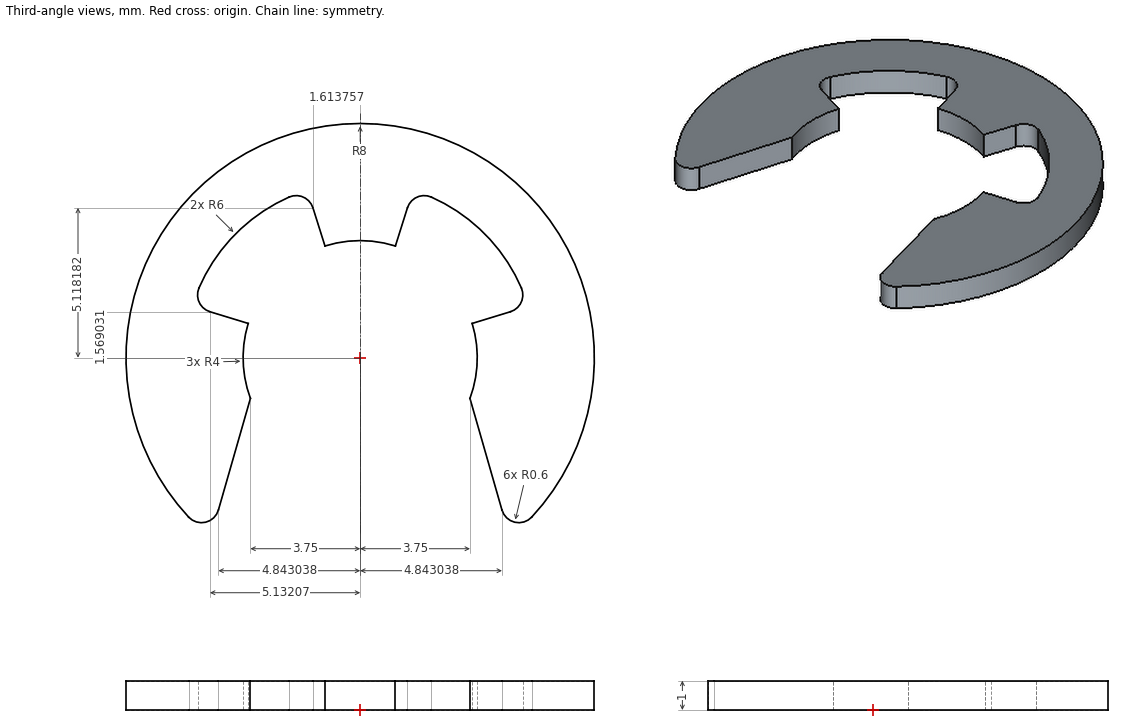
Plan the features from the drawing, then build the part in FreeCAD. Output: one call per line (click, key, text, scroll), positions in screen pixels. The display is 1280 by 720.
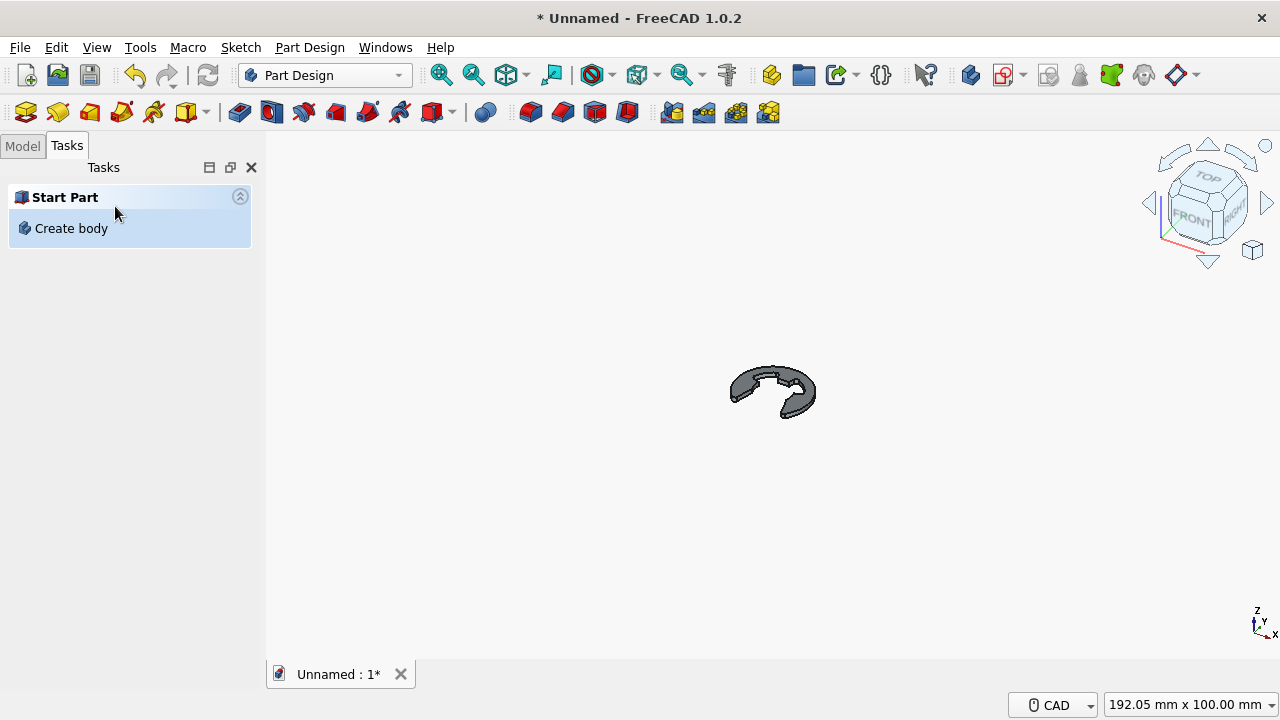
key(0)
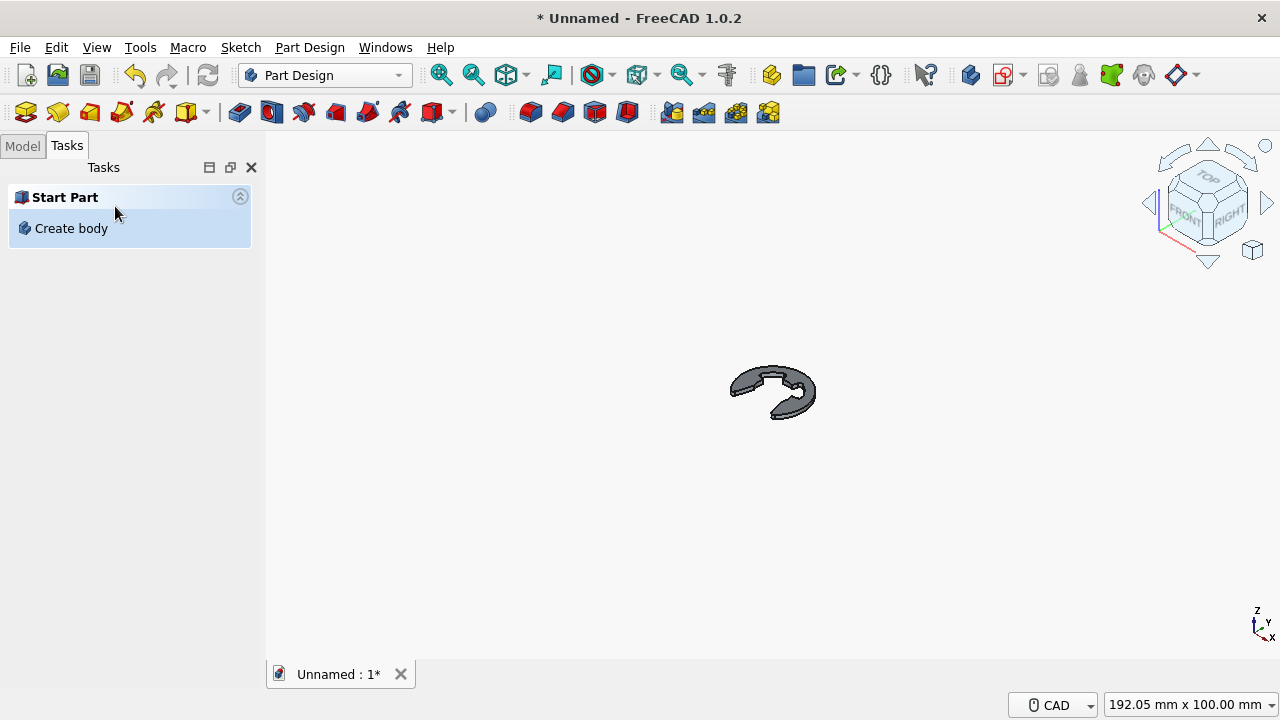
click(442, 76)